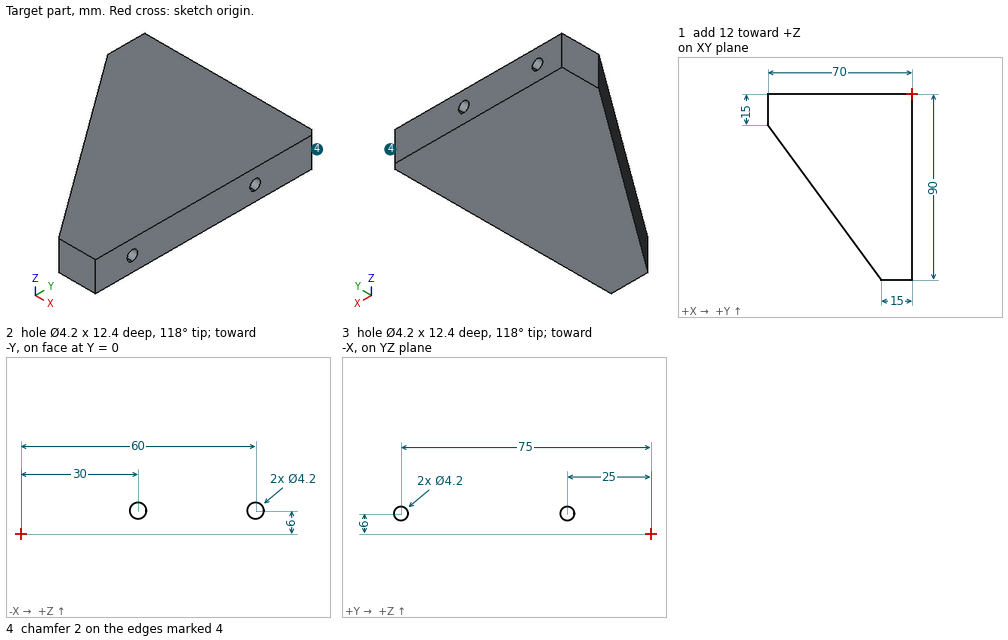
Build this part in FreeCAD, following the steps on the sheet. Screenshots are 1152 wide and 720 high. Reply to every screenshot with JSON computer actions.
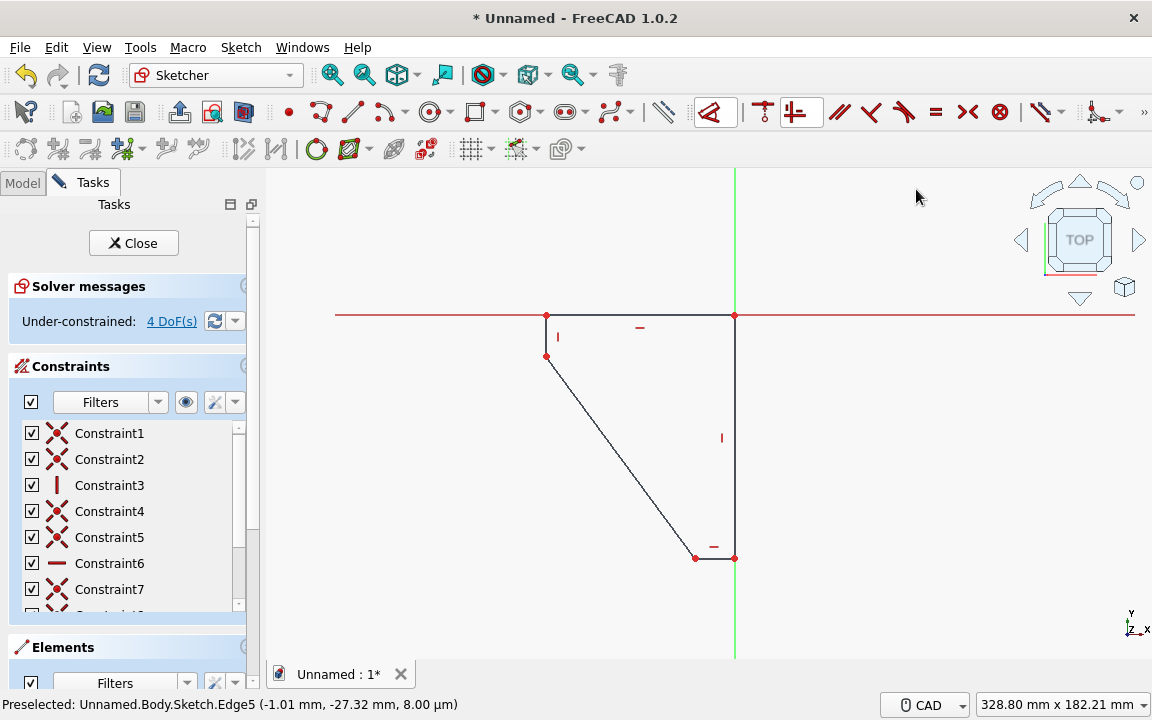
{"action": "left_click", "coordinate": [678, 315]}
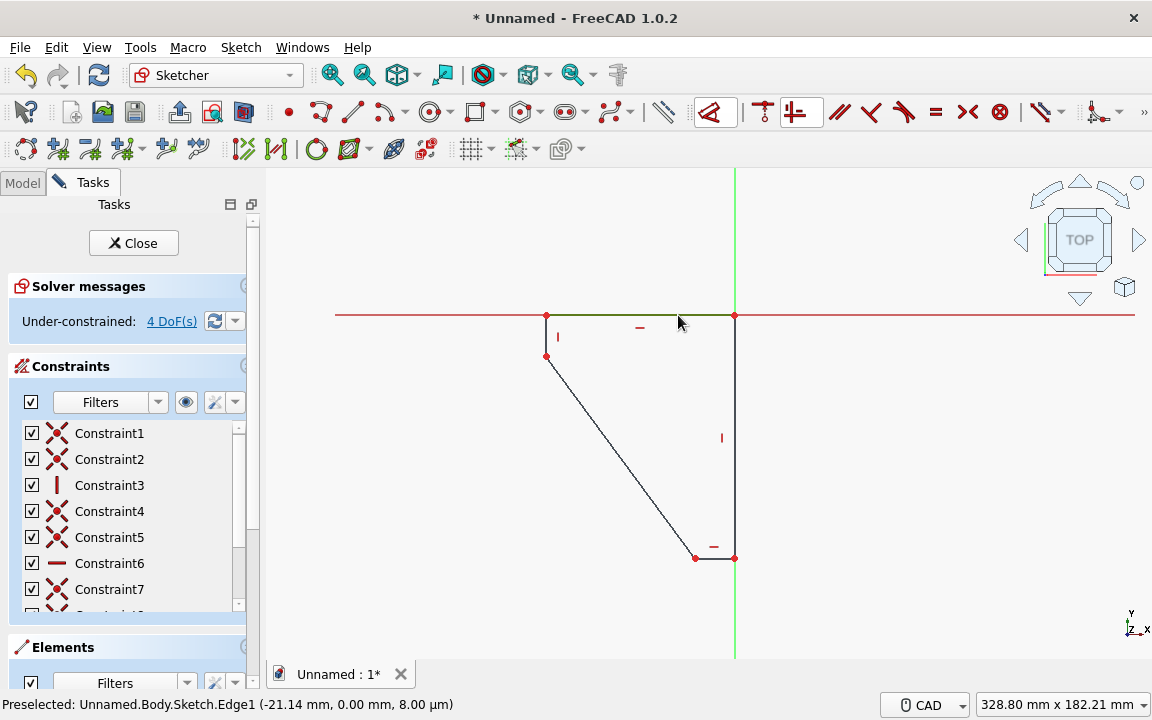
{"action": "key", "text": "l"}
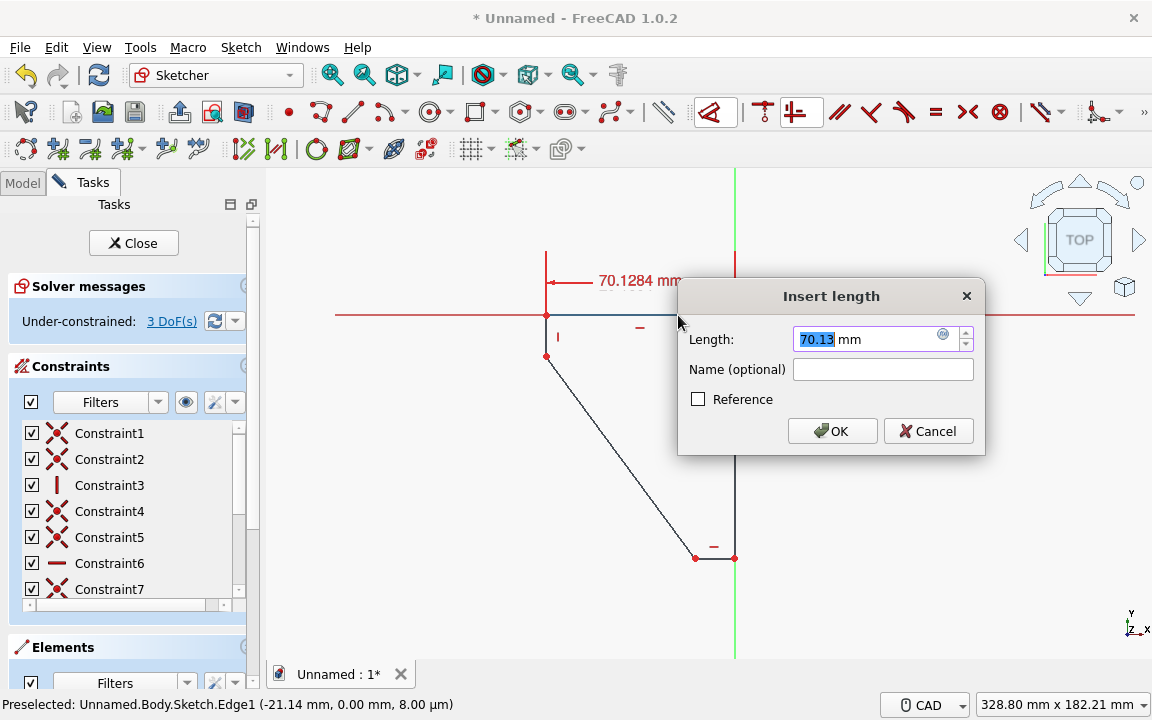
{"action": "type", "text": "70"}
{"action": "key", "text": "Return"}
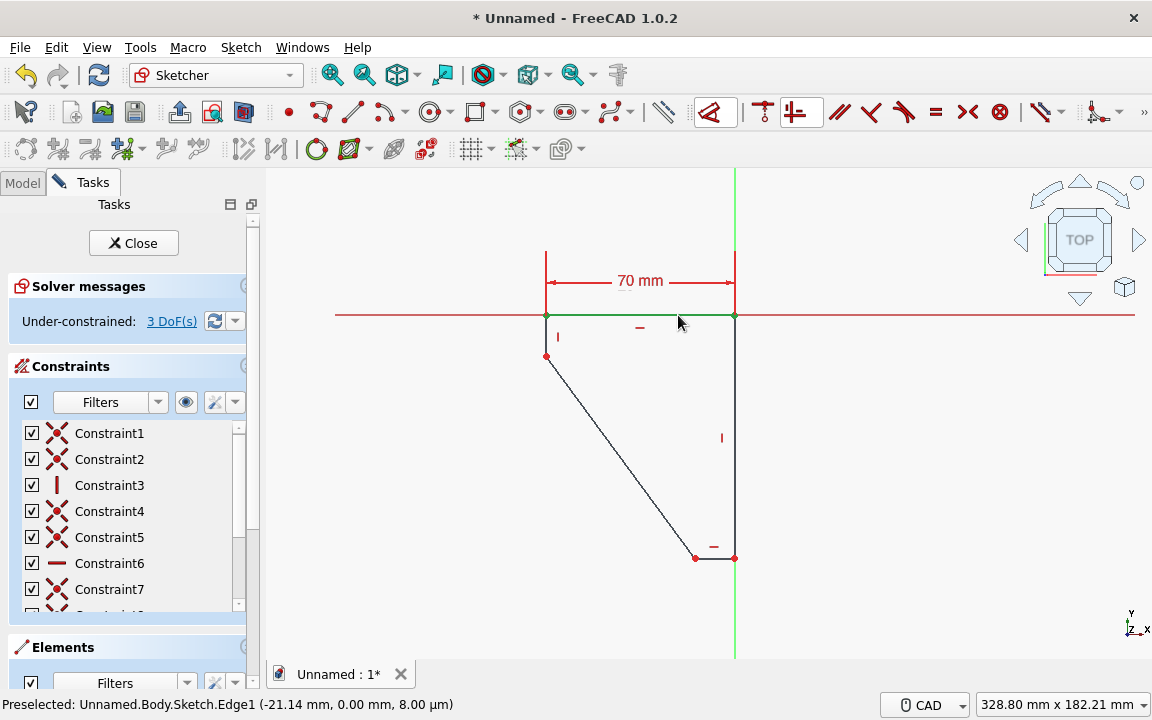
{"action": "left_click", "coordinate": [546, 328]}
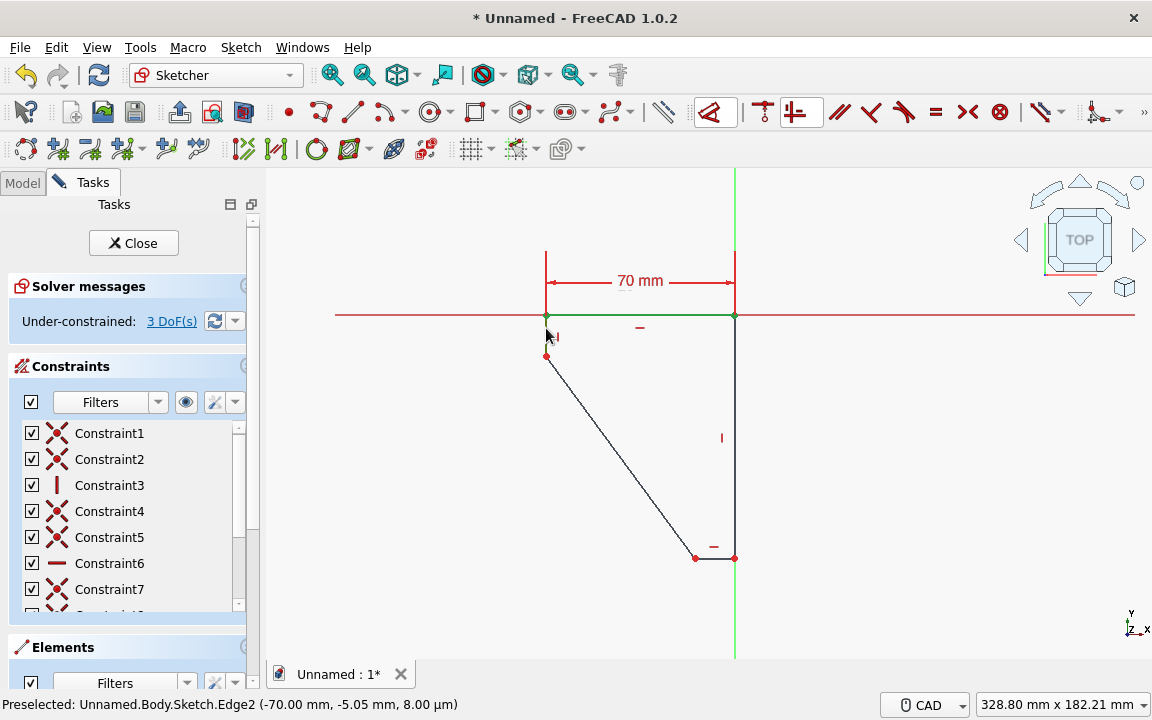
{"action": "key", "text": "i"}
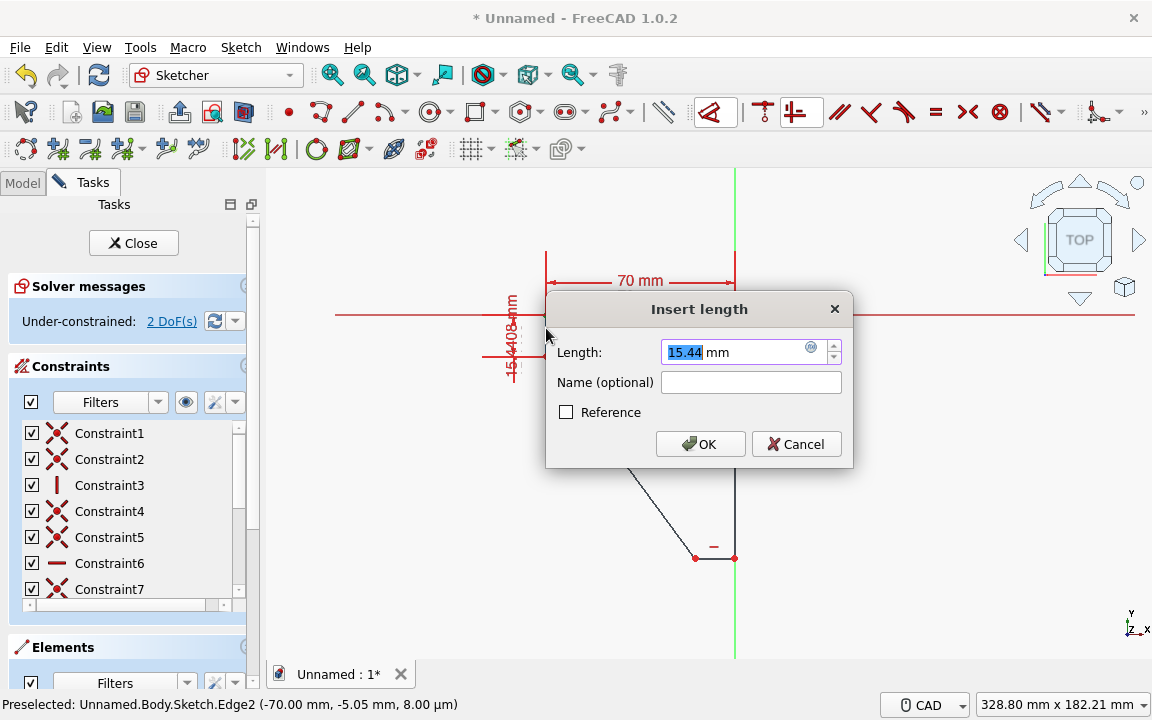
{"action": "type", "text": "15"}
{"action": "key", "text": "Return"}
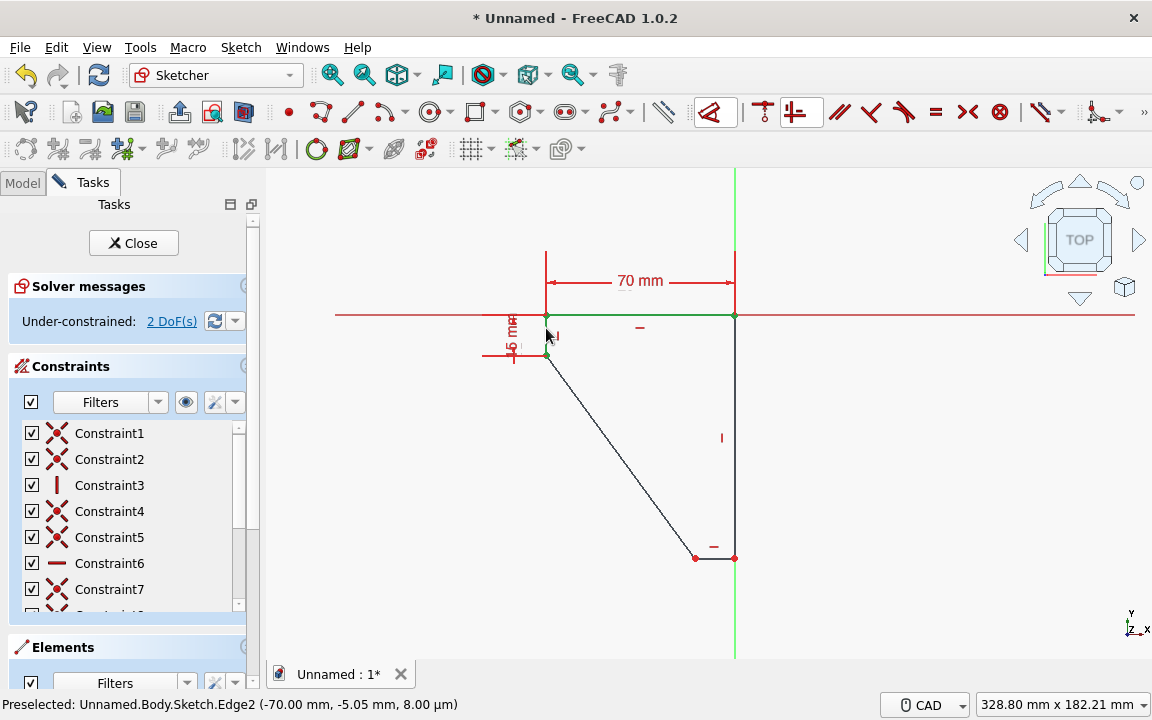
{"action": "left_click", "coordinate": [707, 559]}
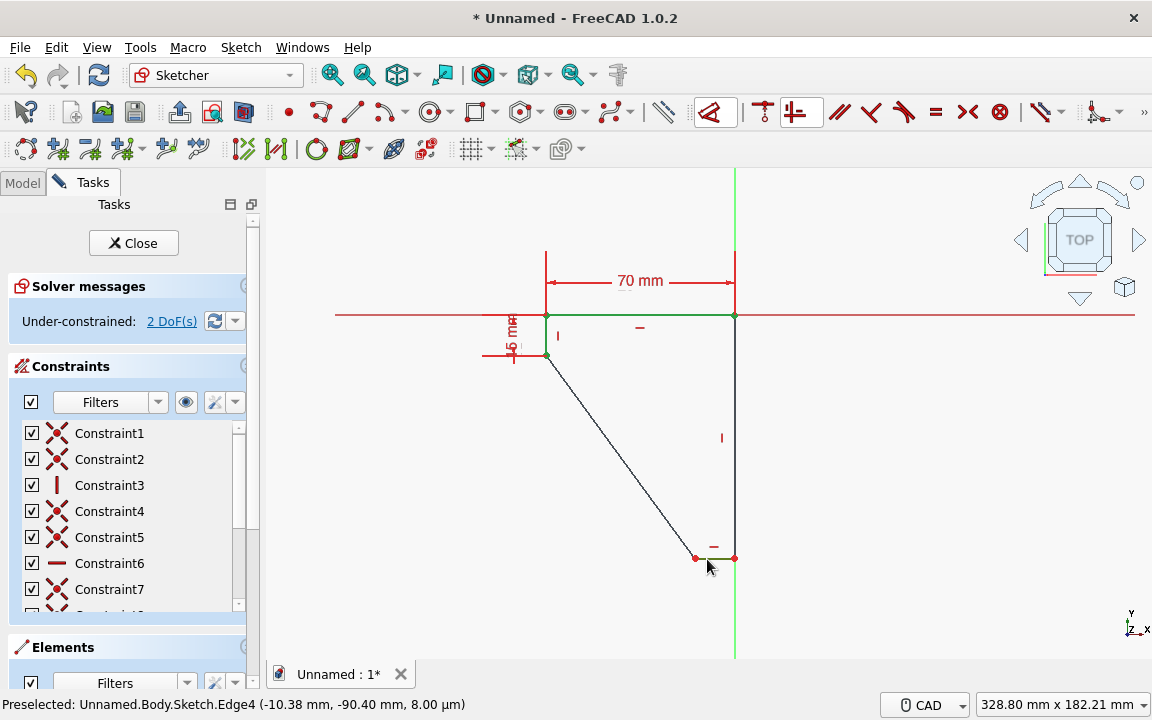
{"action": "key", "text": "l"}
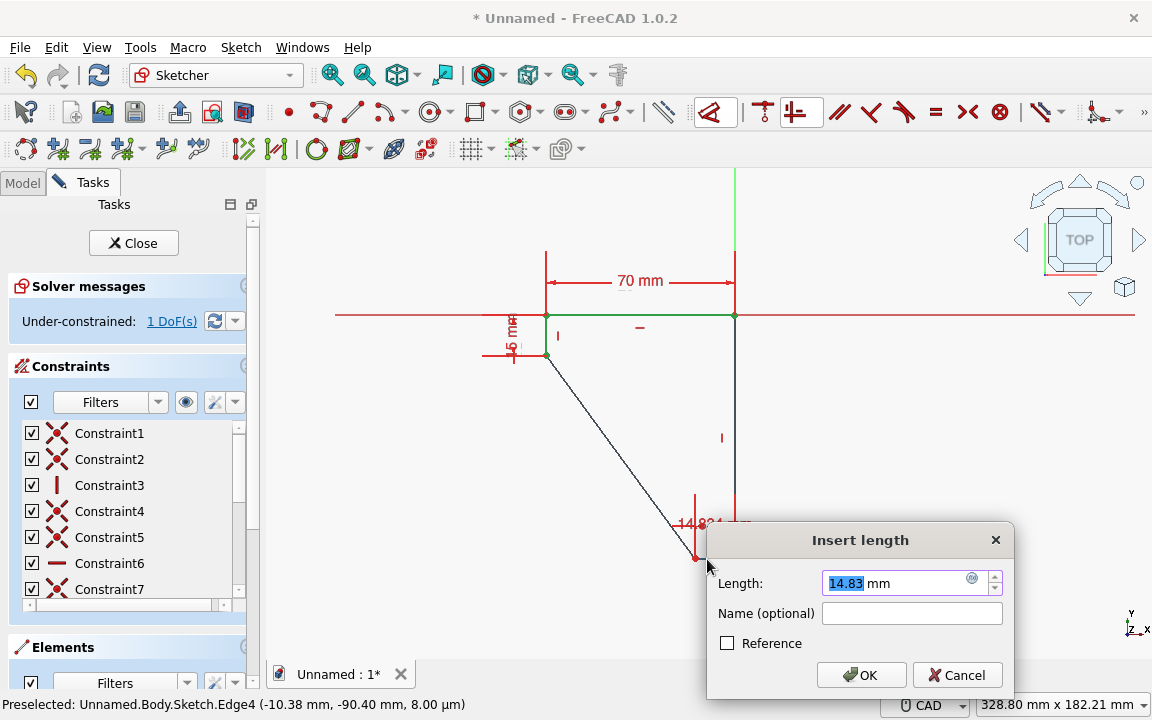
{"action": "type", "text": "15"}
{"action": "key", "text": "Return"}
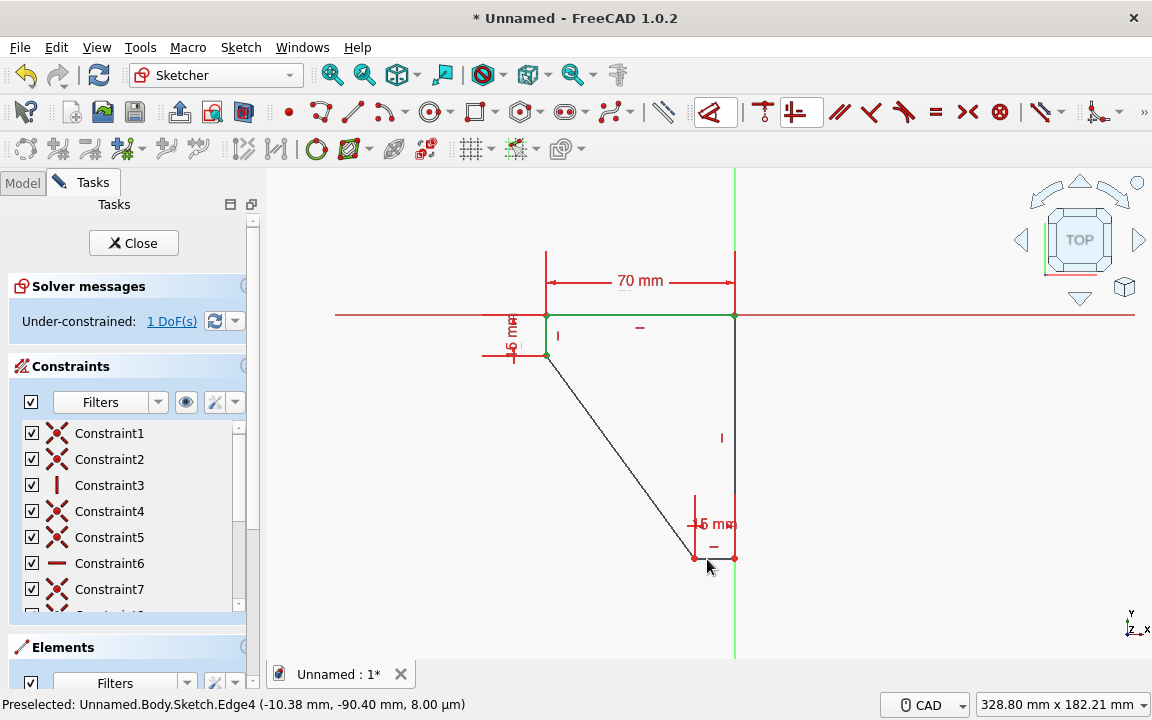
{"action": "left_click", "coordinate": [735, 486]}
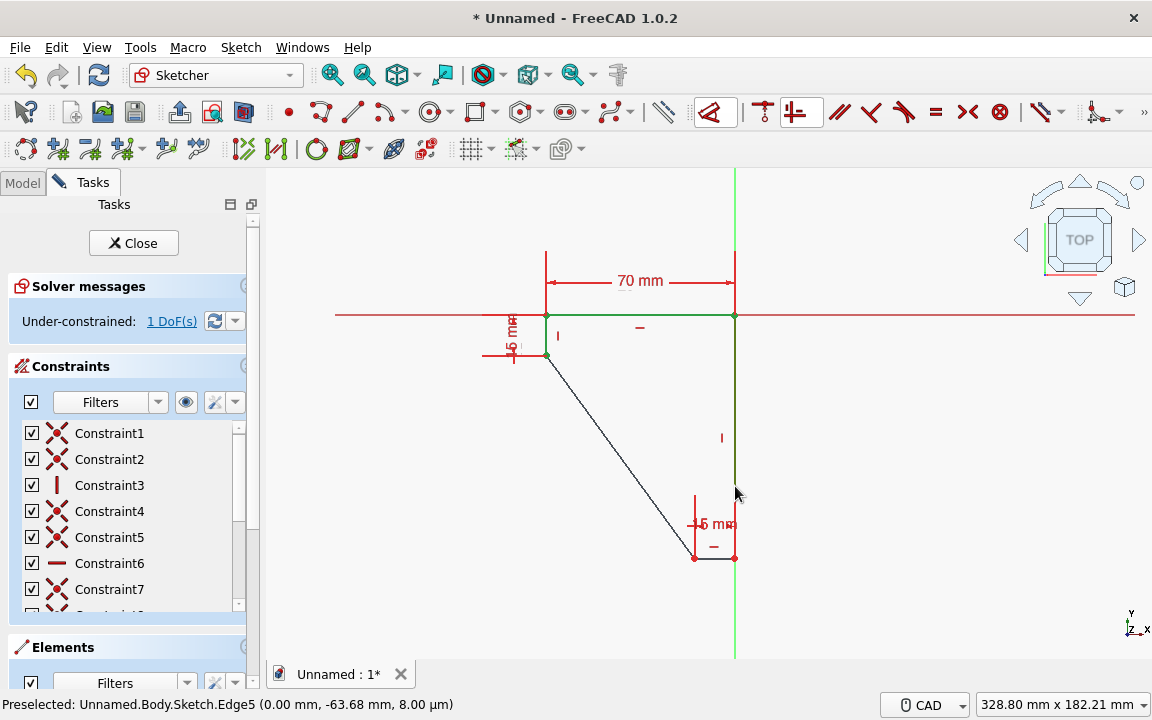
{"action": "key", "text": "i"}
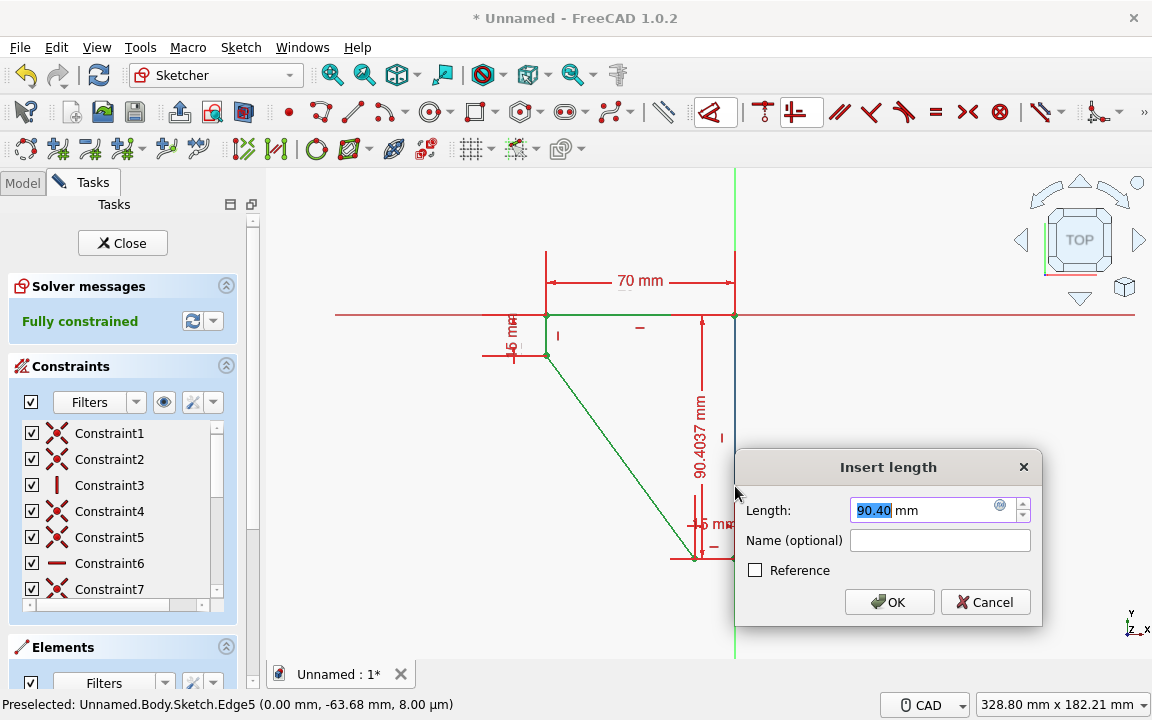
{"action": "type", "text": "90"}
{"action": "key", "text": "Return"}